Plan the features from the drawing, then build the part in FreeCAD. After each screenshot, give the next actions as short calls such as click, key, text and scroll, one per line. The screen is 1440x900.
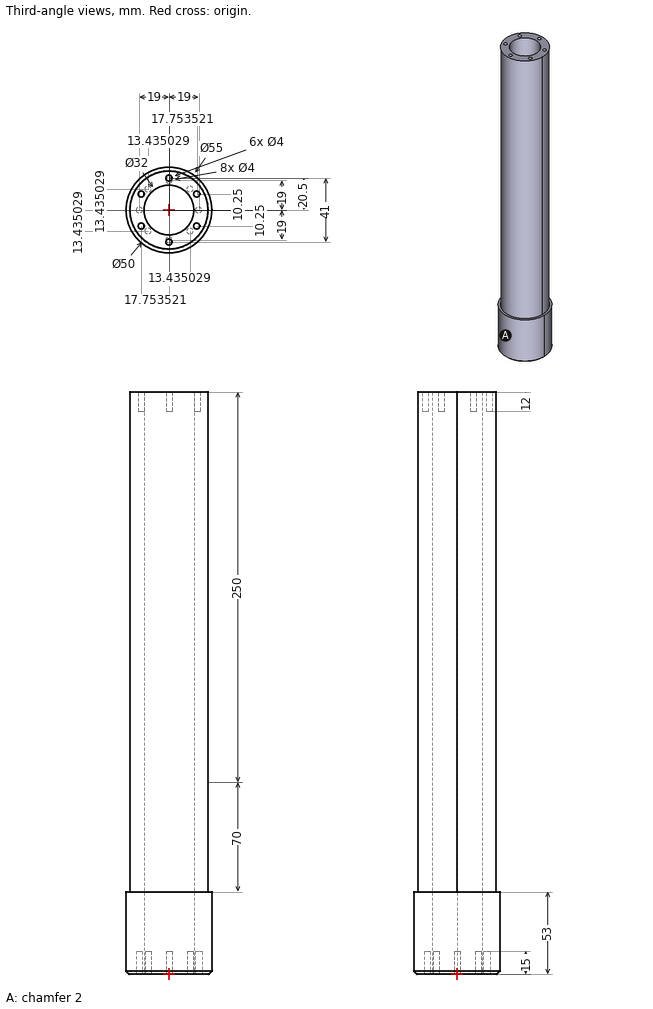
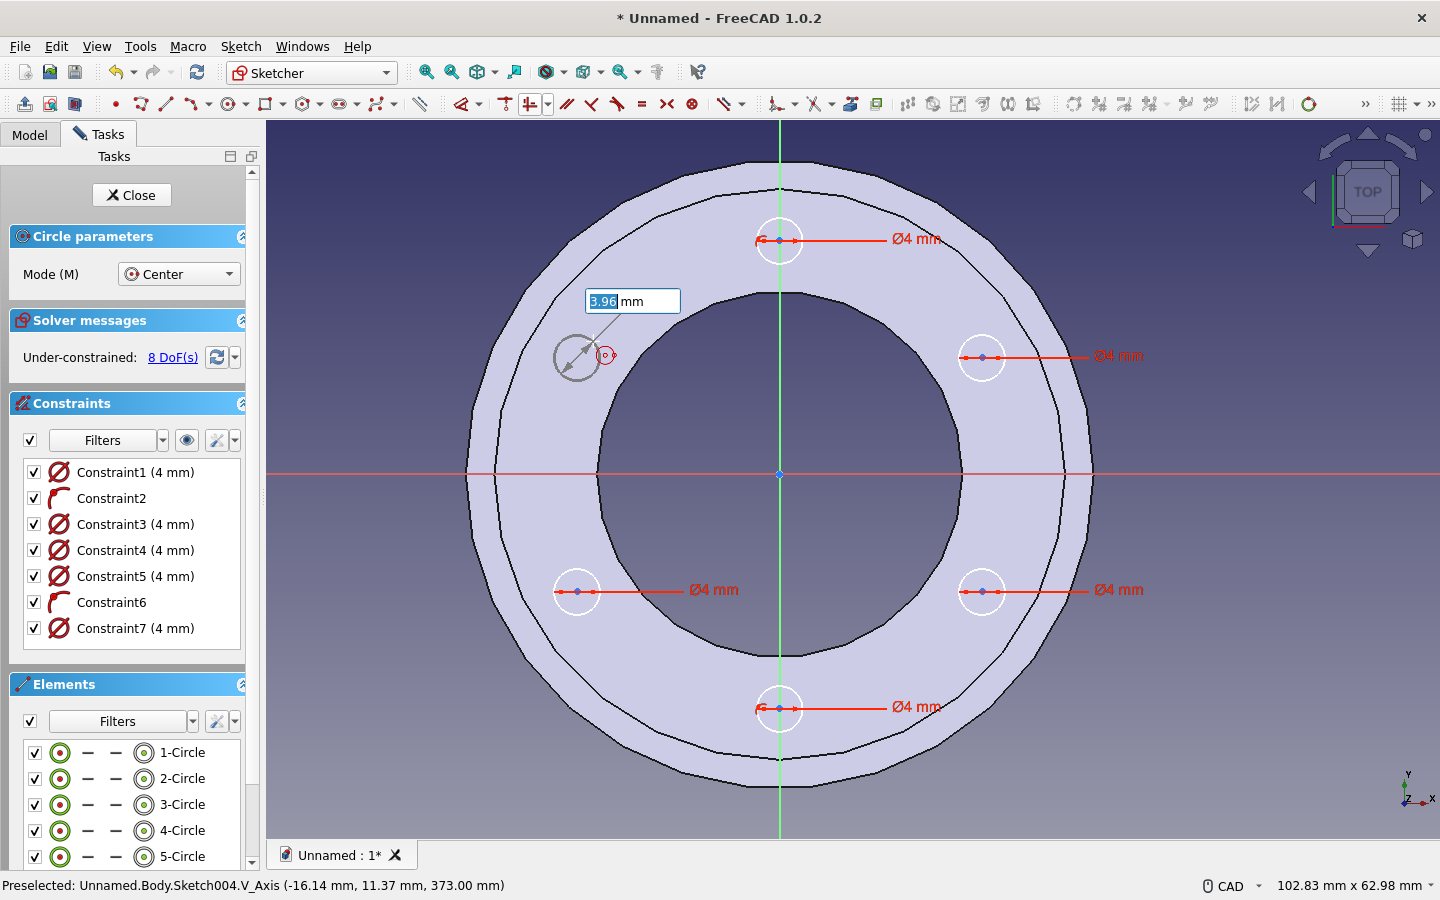
text(4)
key(Return)
key(Escape)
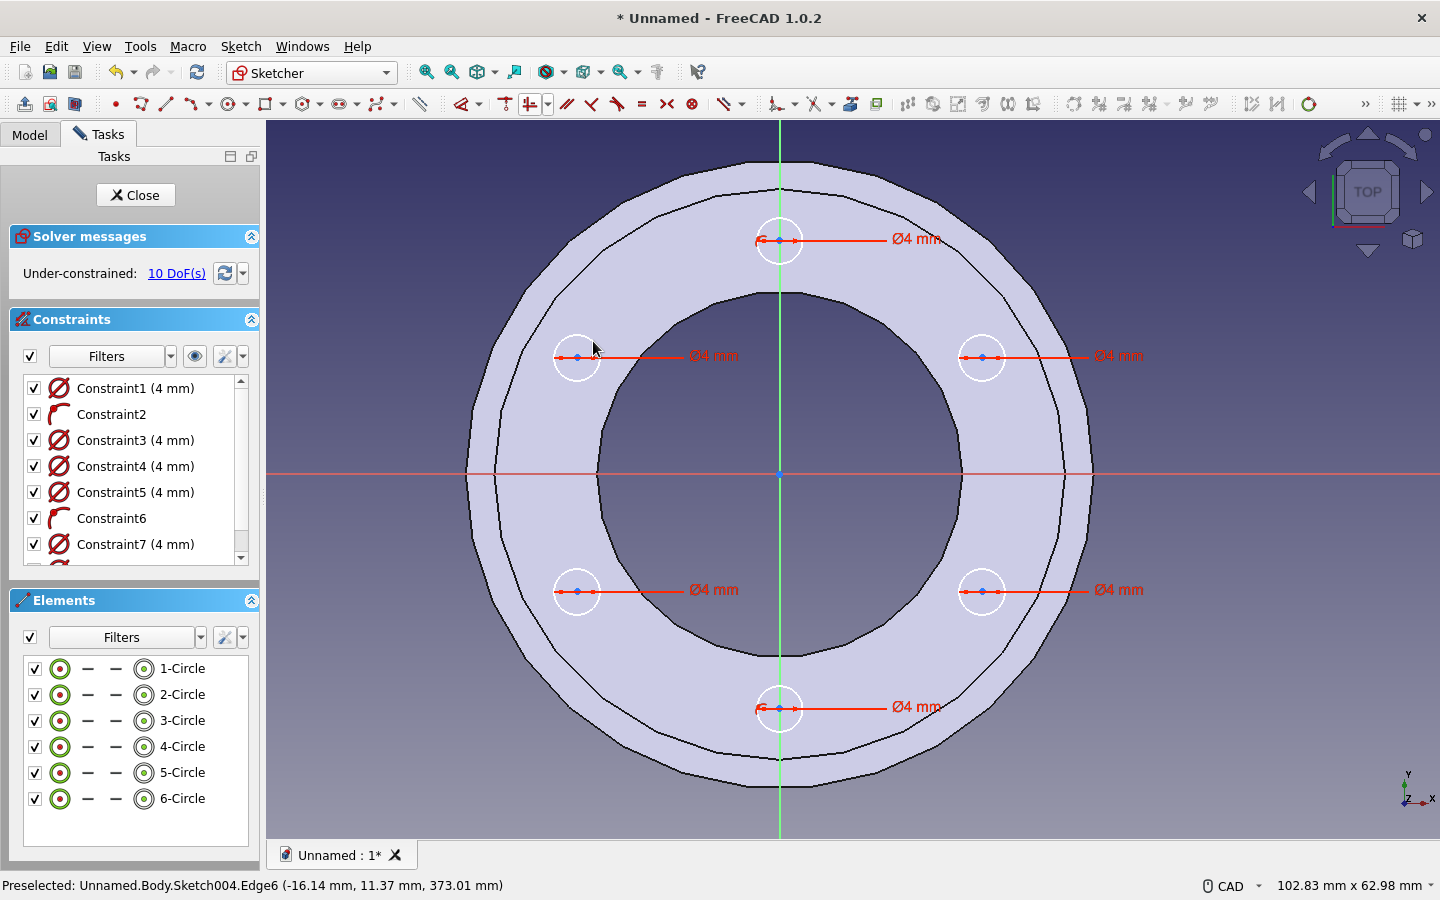
click(982, 358)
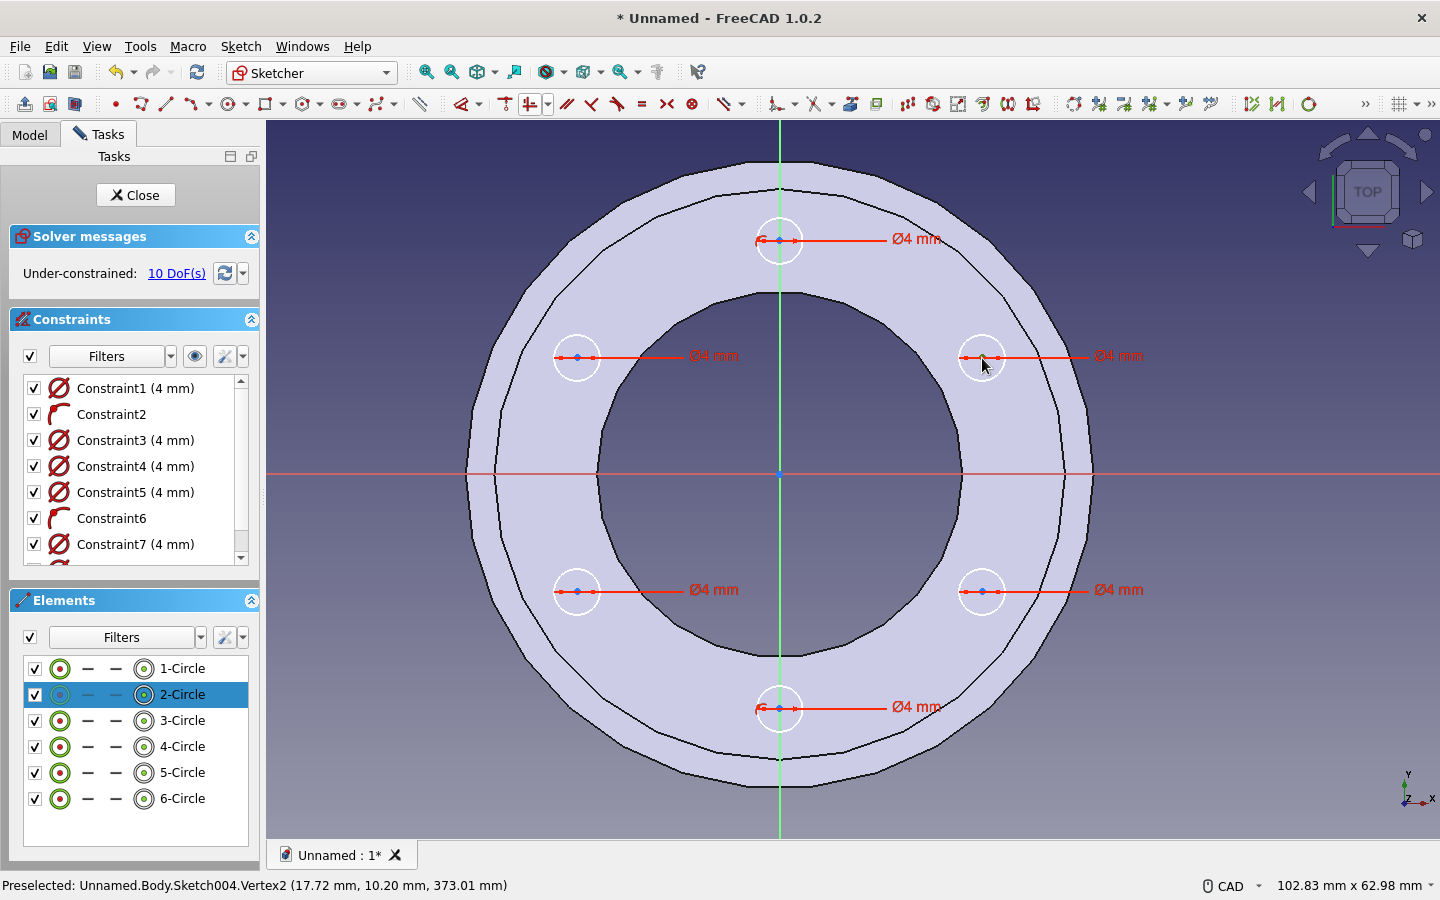
click(982, 592)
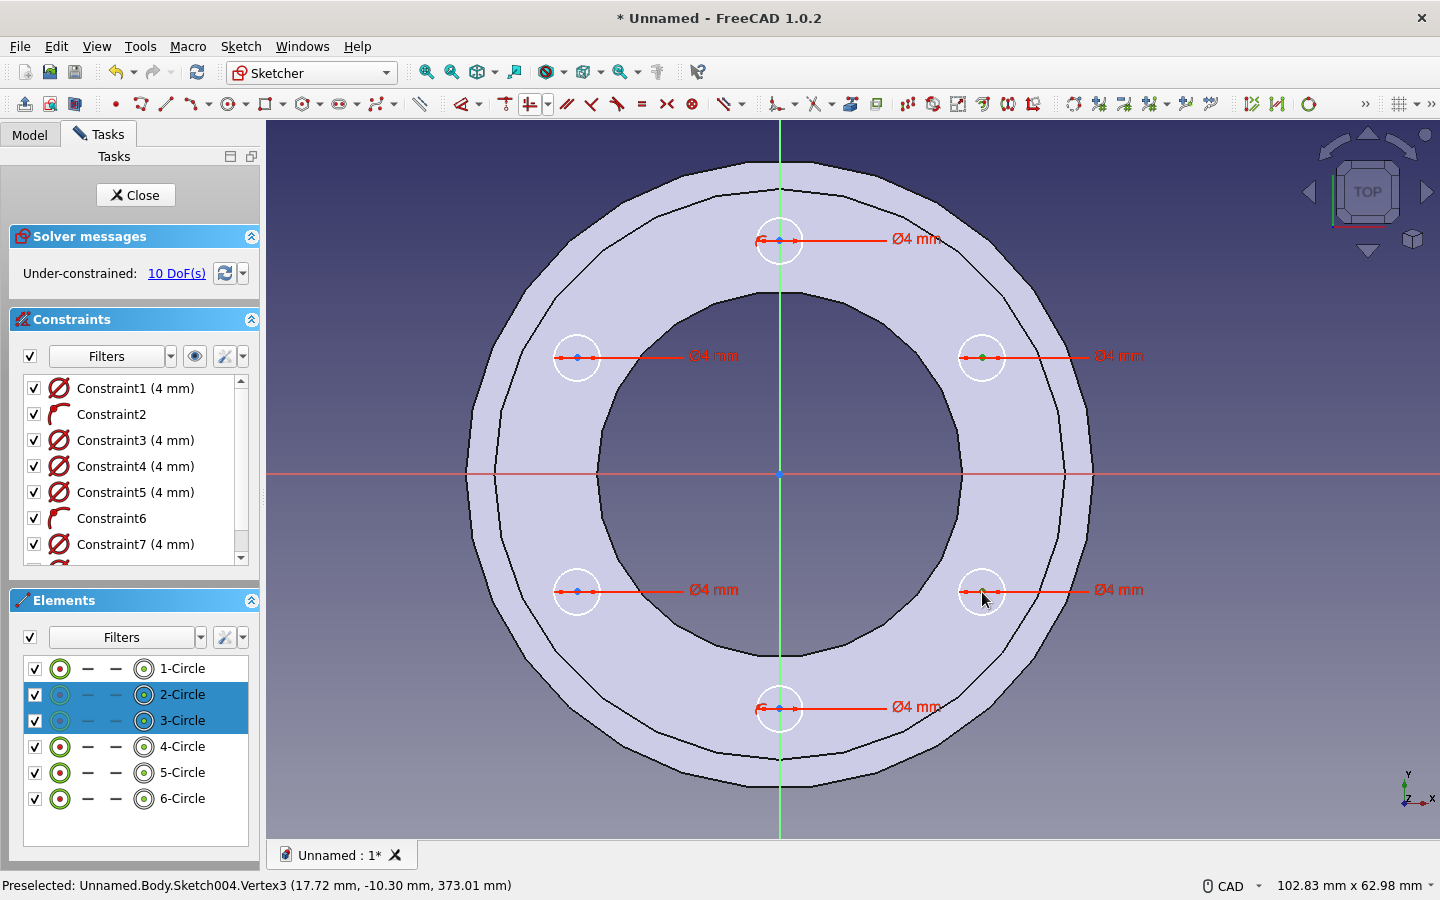
click(548, 104)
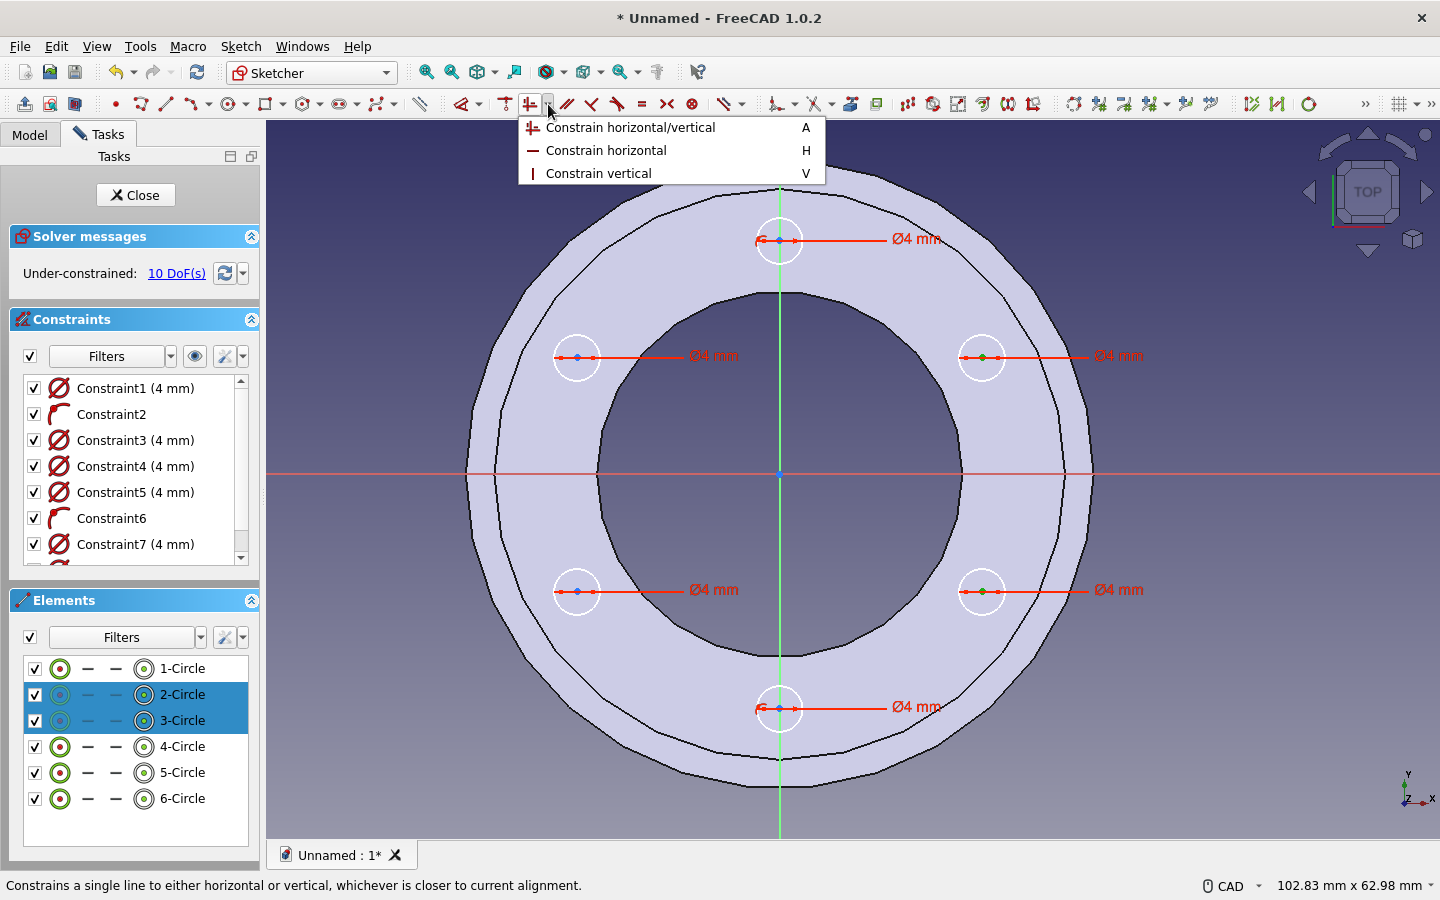
click(672, 174)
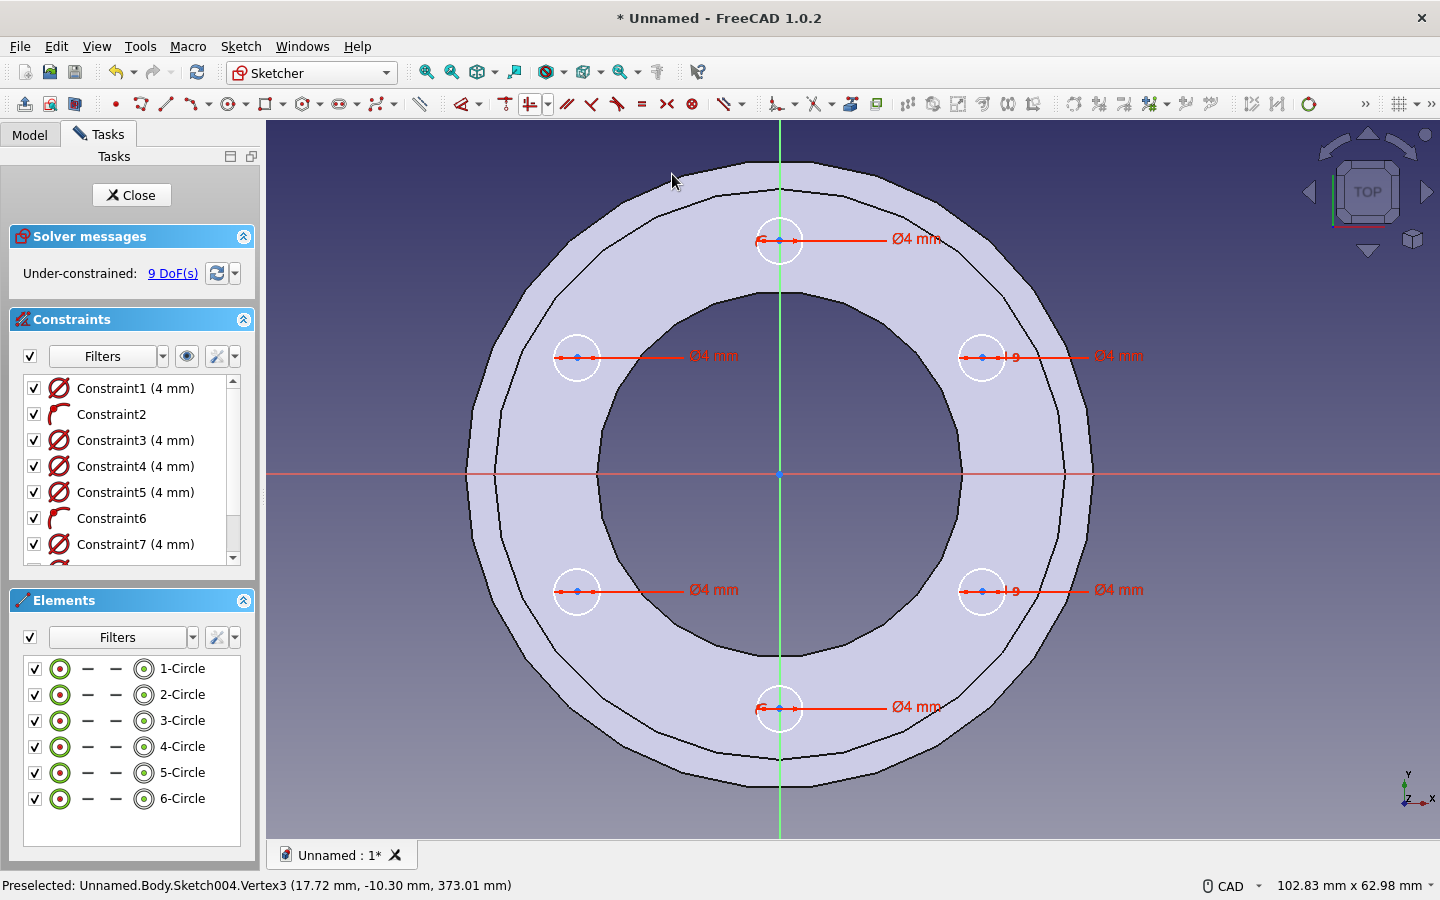
click(982, 592)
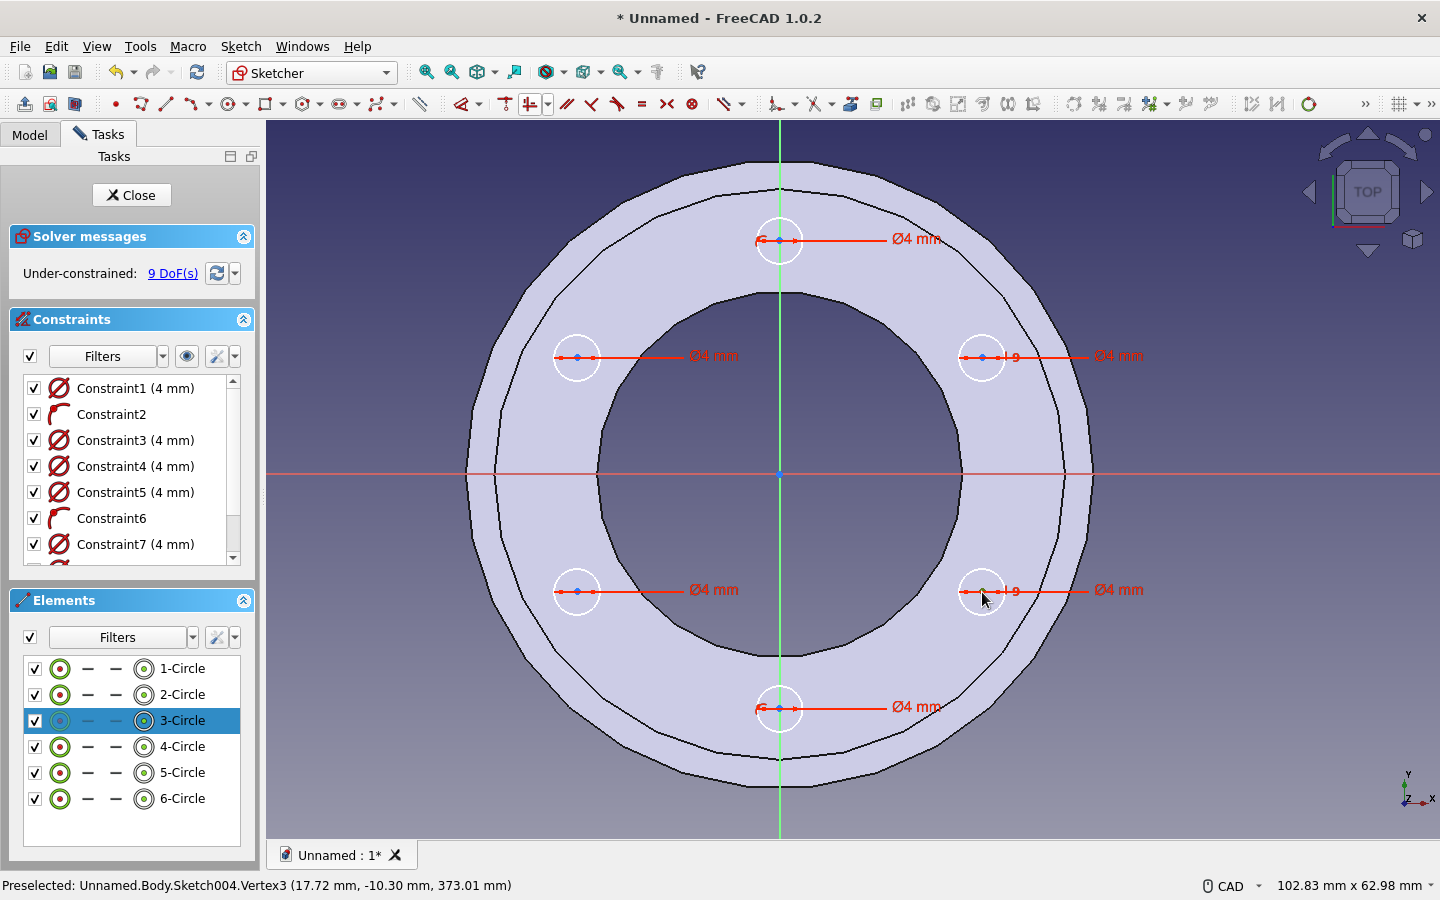
click(577, 592)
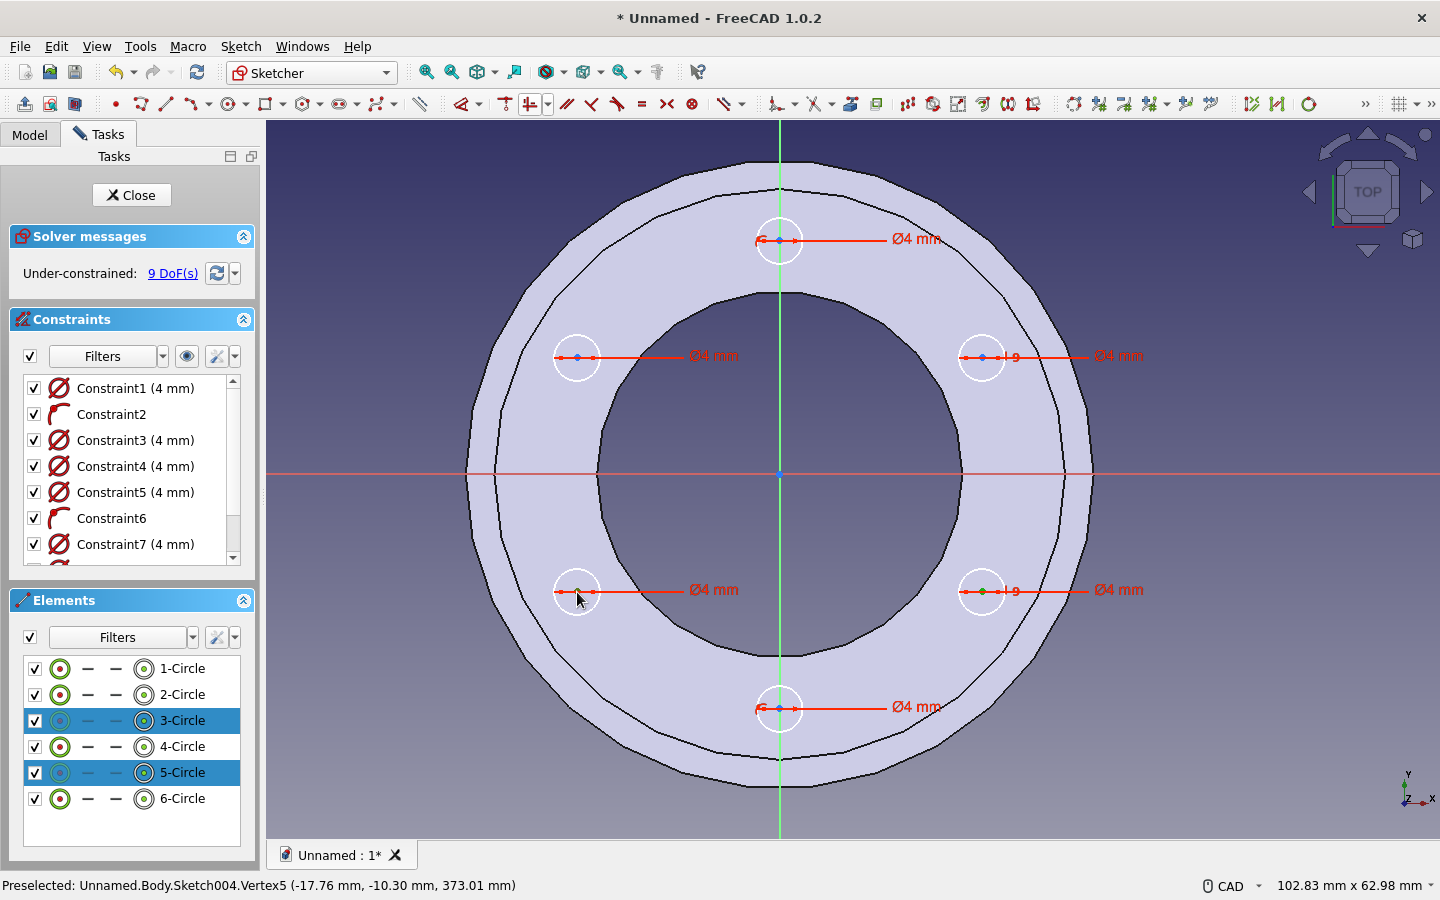
click(548, 104)